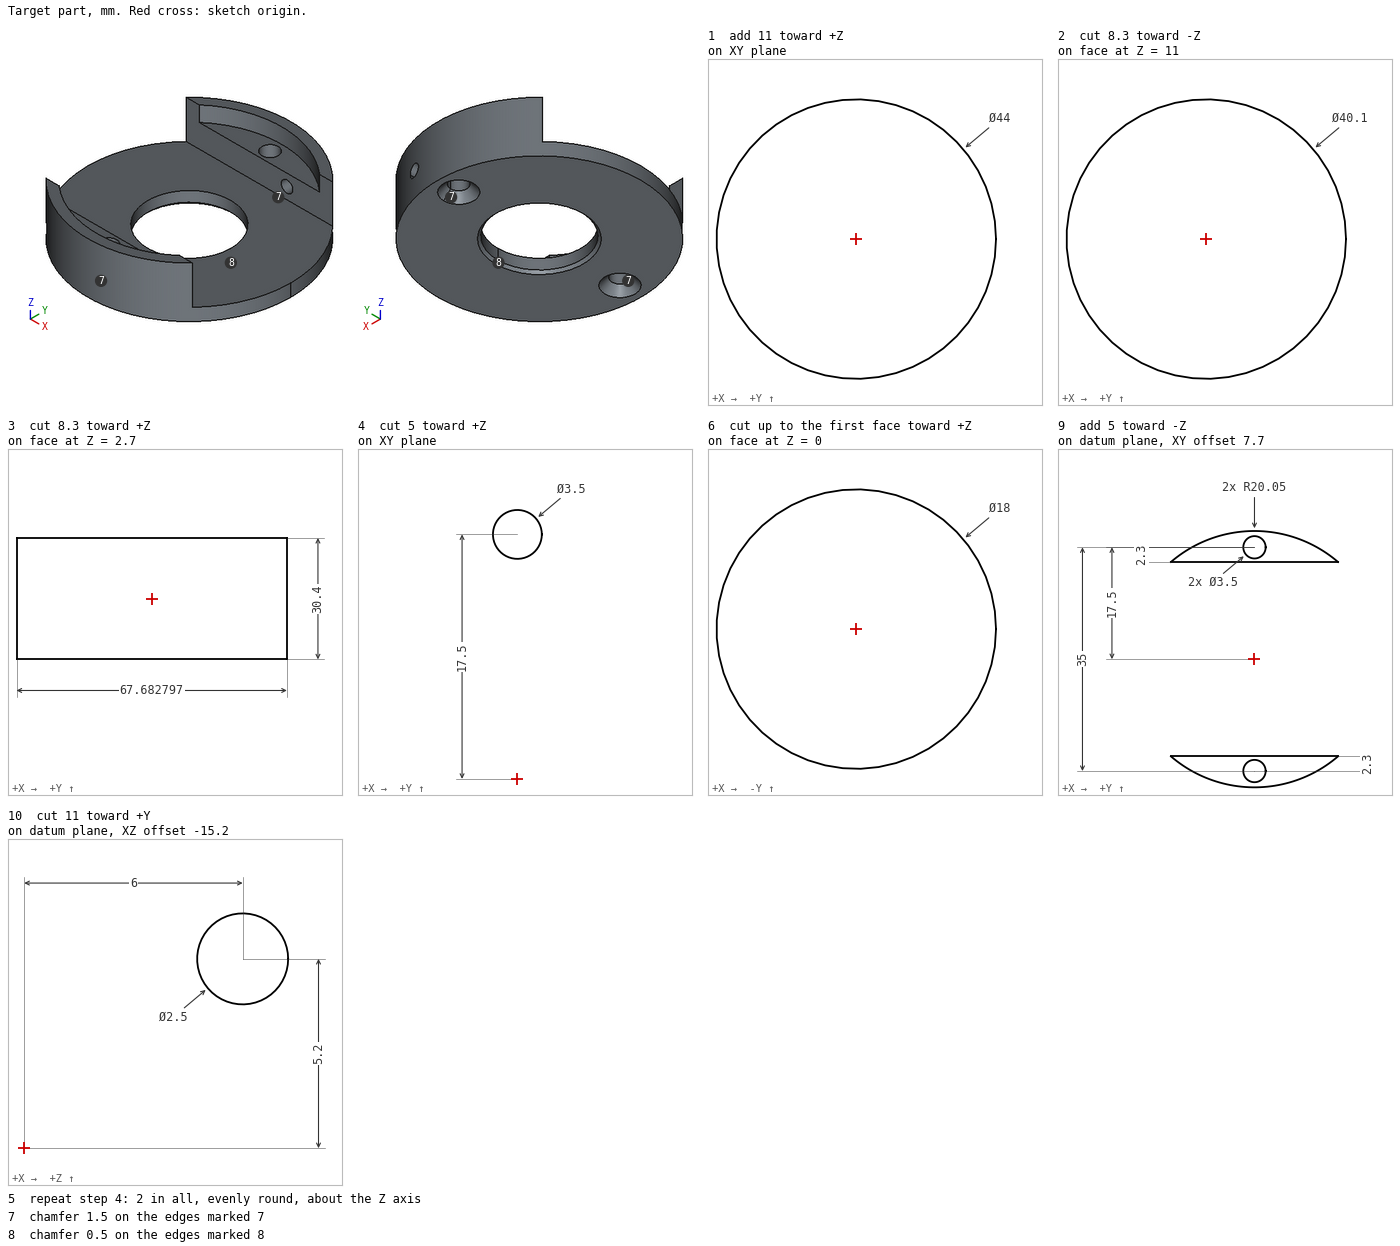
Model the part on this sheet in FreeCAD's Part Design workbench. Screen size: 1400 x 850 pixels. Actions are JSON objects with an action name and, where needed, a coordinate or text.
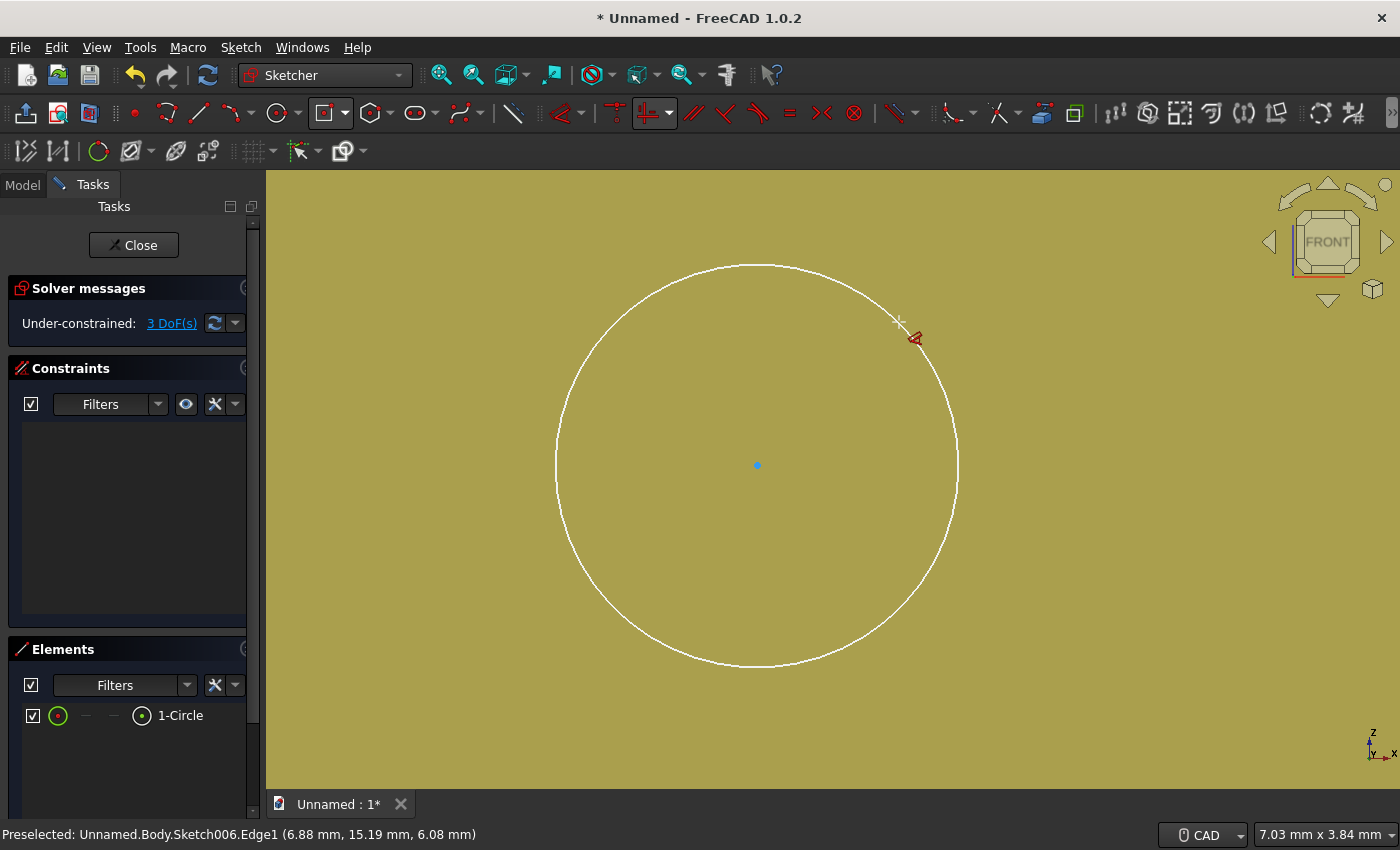
{"action": "left_click", "coordinate": [899, 323]}
{"action": "left_click", "coordinate": [922, 300]}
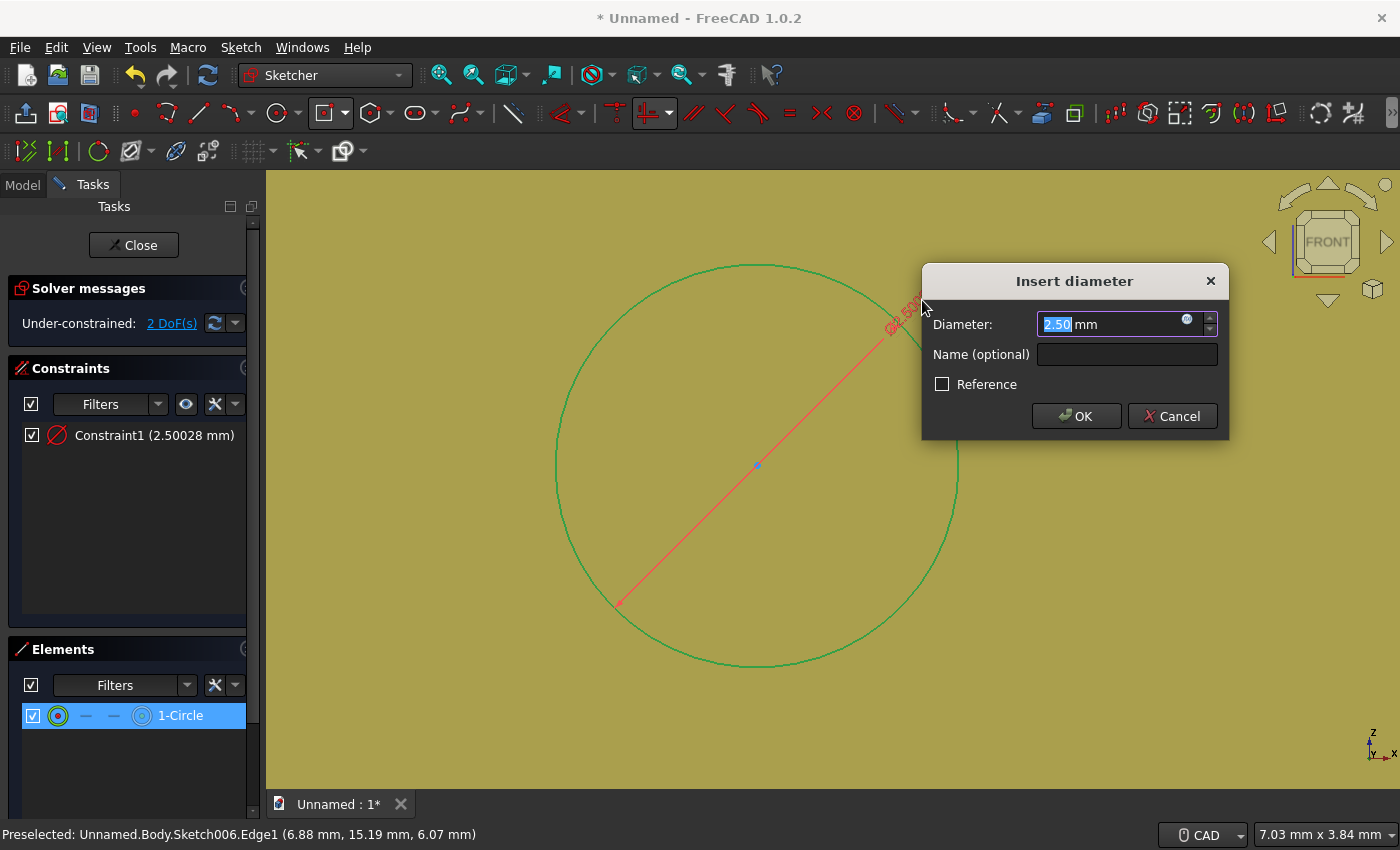
{"action": "type", "text": "2.5"}
{"action": "key", "text": "Return"}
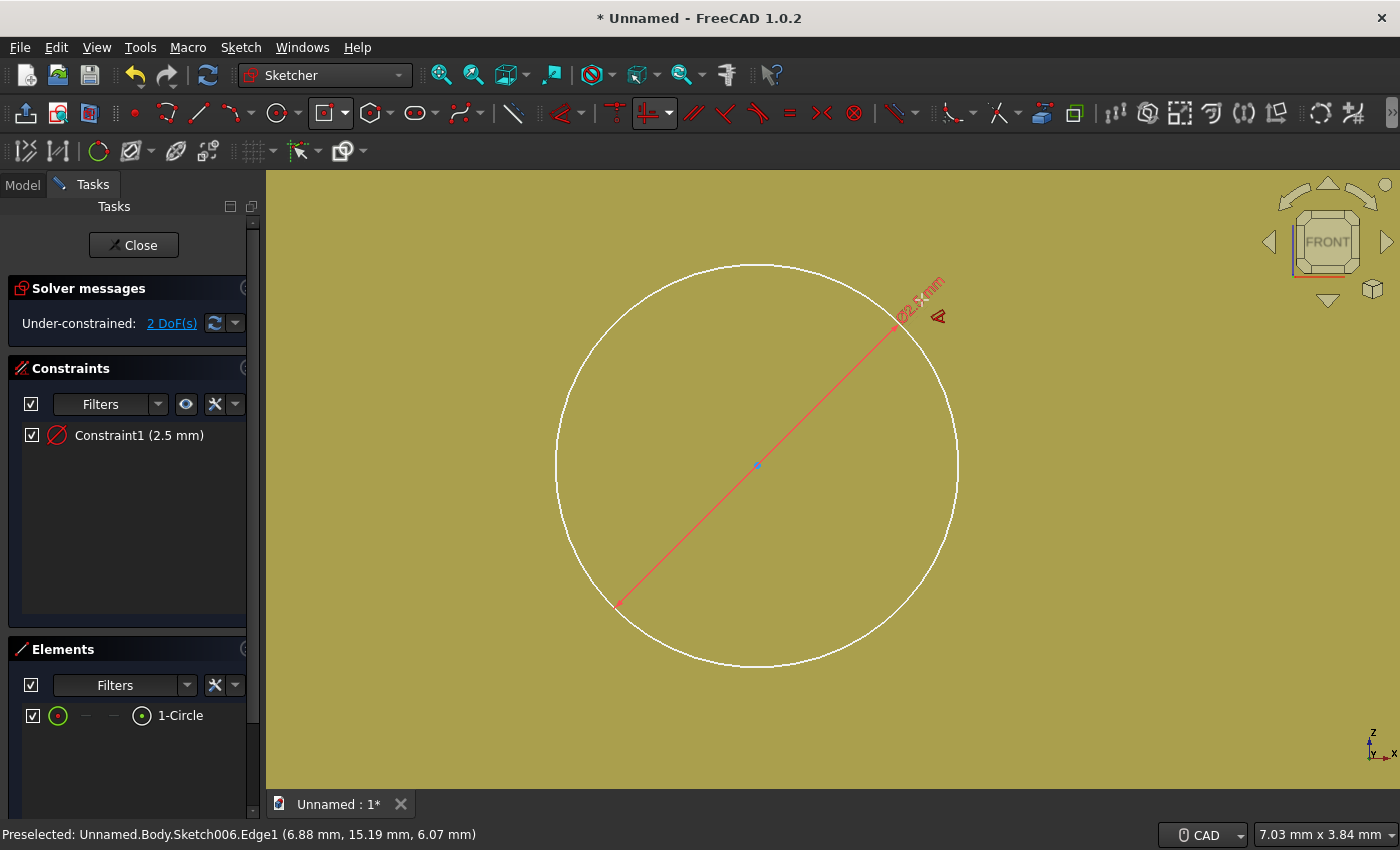
{"action": "left_click", "coordinate": [757, 466]}
{"action": "left_click", "coordinate": [526, 432]}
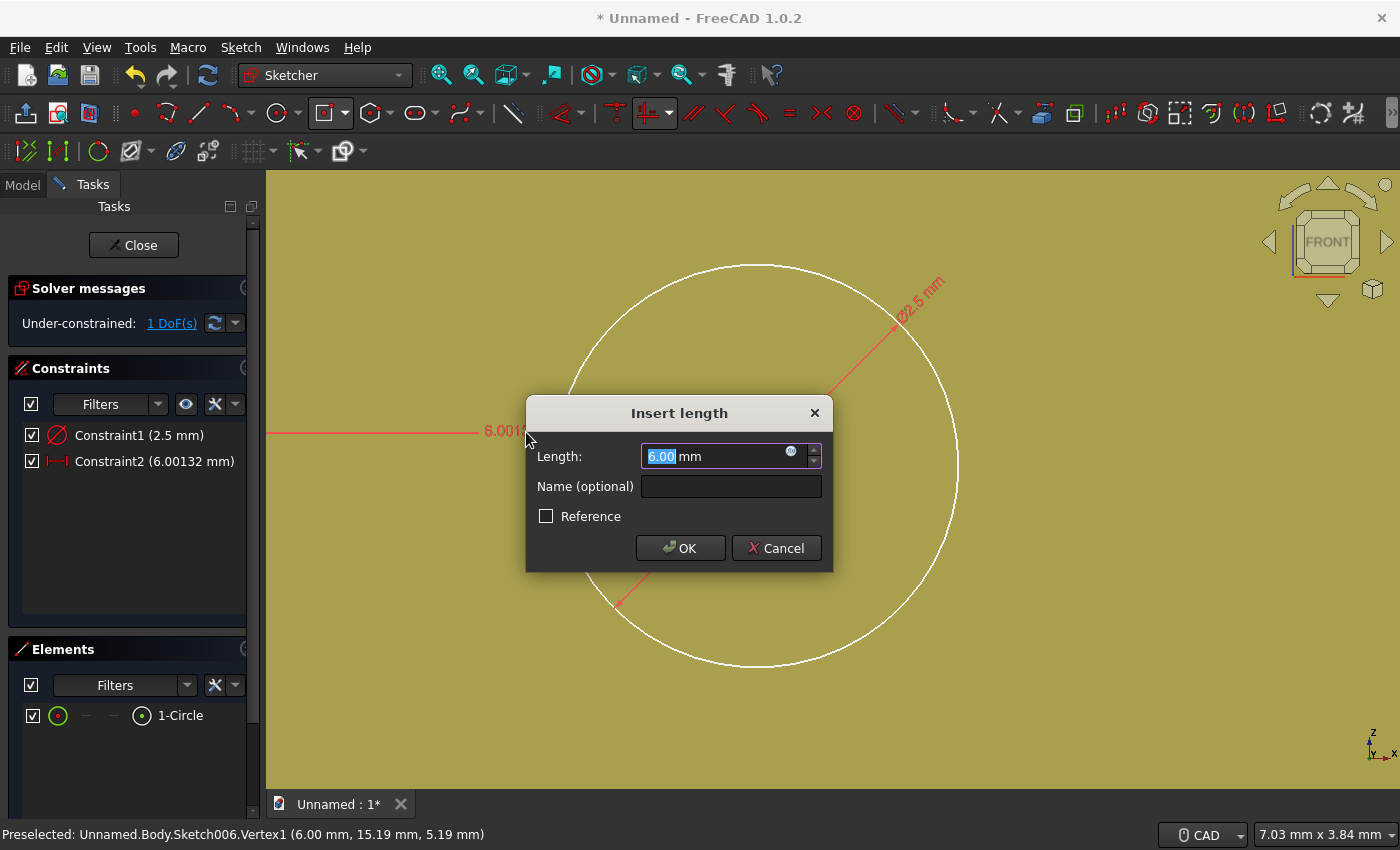
{"action": "type", "text": "6"}
{"action": "key", "text": "Return"}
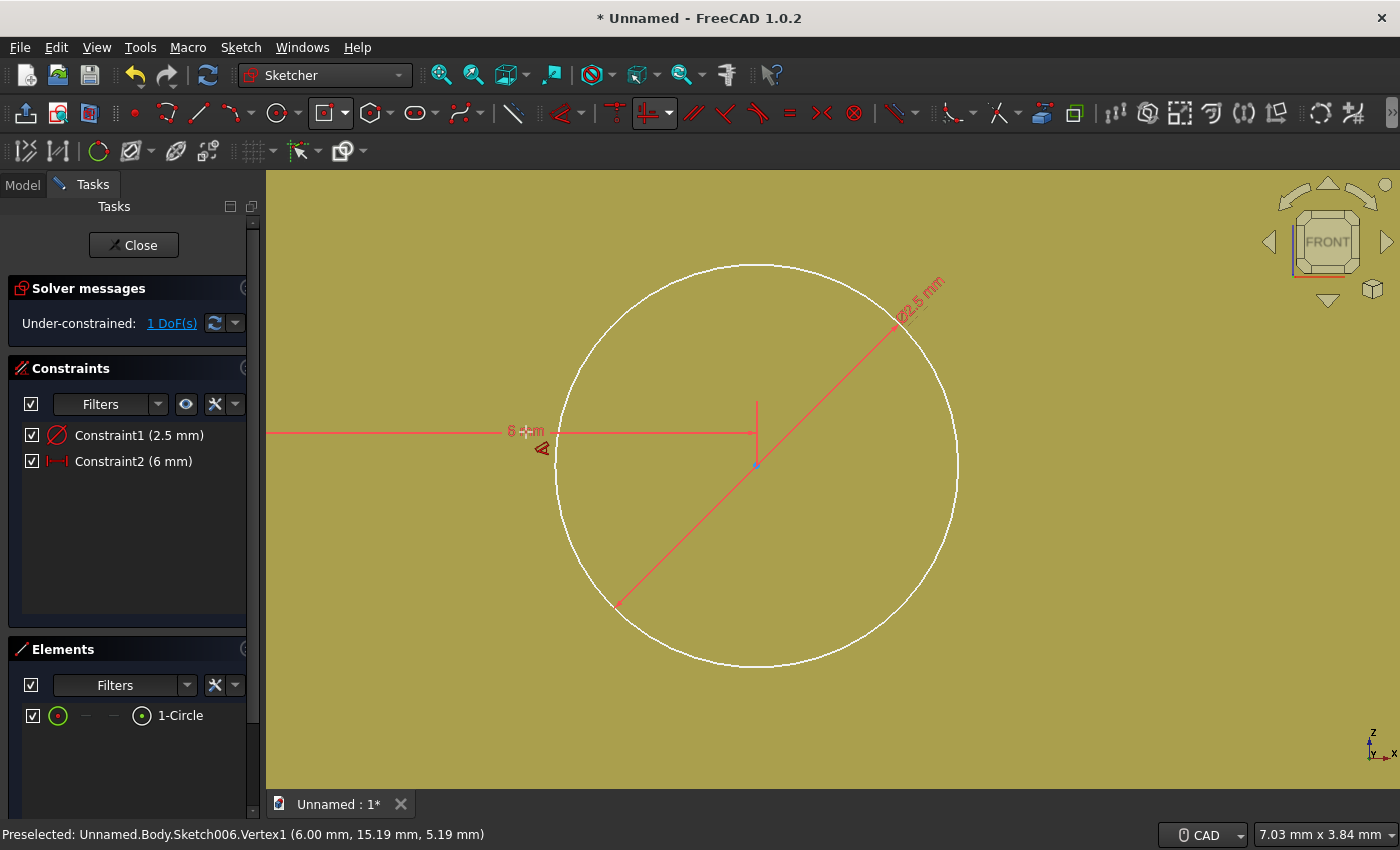
{"action": "left_click", "coordinate": [757, 466]}
{"action": "left_click", "coordinate": [791, 613]}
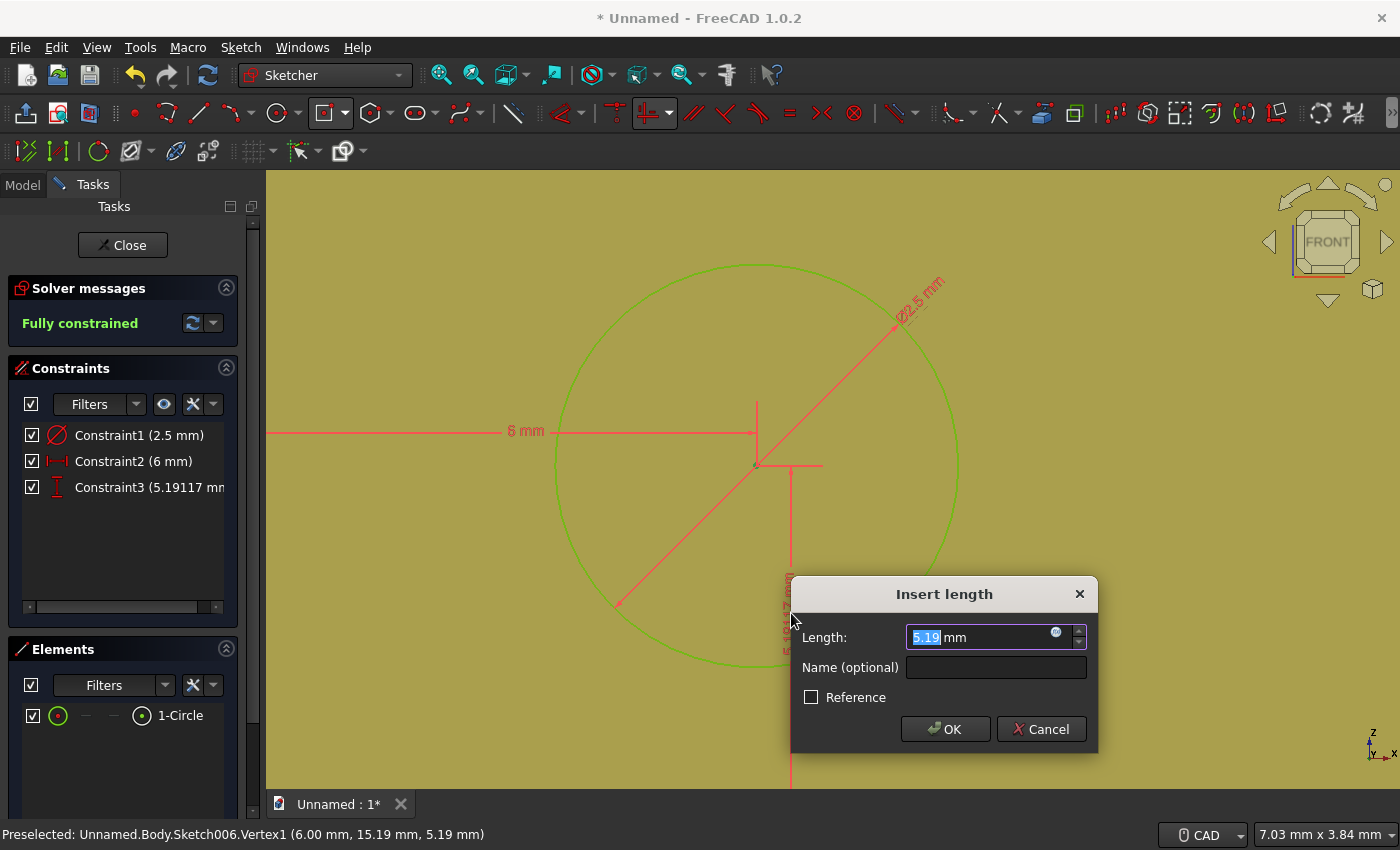
{"action": "type", "text": "5.2"}
{"action": "key", "text": "Return"}
{"action": "key", "text": "Escape"}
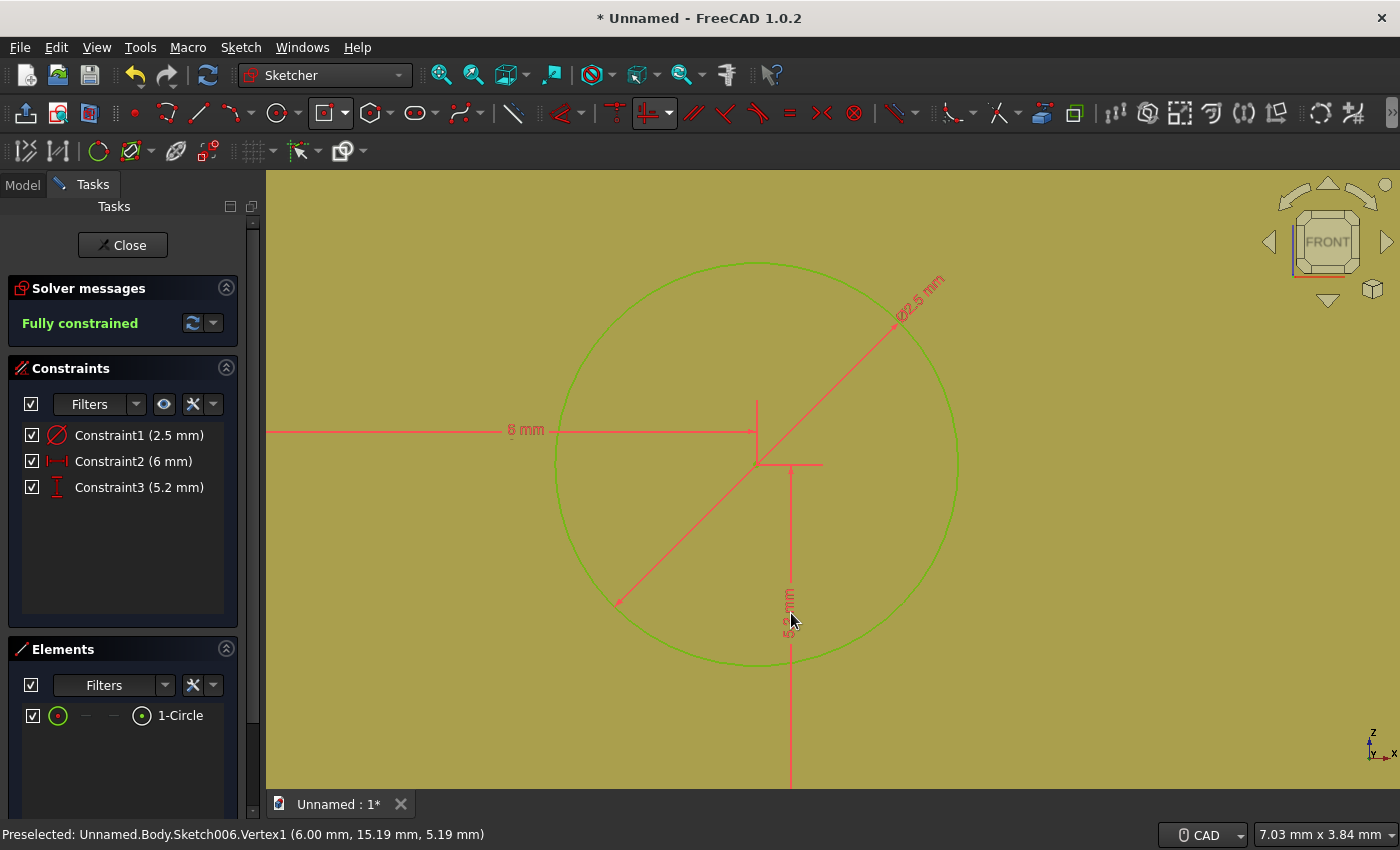
{"action": "left_click", "coordinate": [123, 245]}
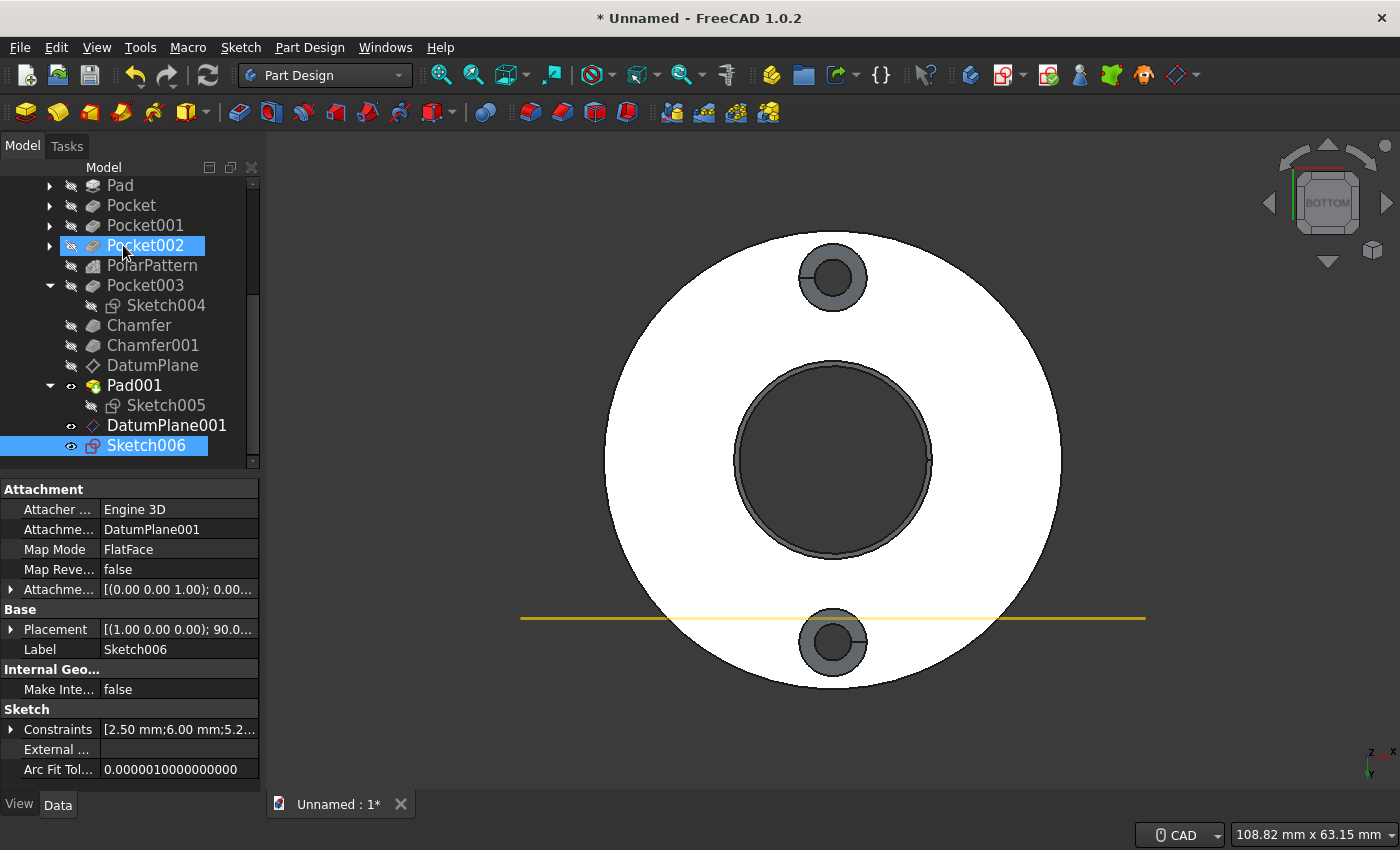
{"action": "left_click", "coordinate": [240, 112]}